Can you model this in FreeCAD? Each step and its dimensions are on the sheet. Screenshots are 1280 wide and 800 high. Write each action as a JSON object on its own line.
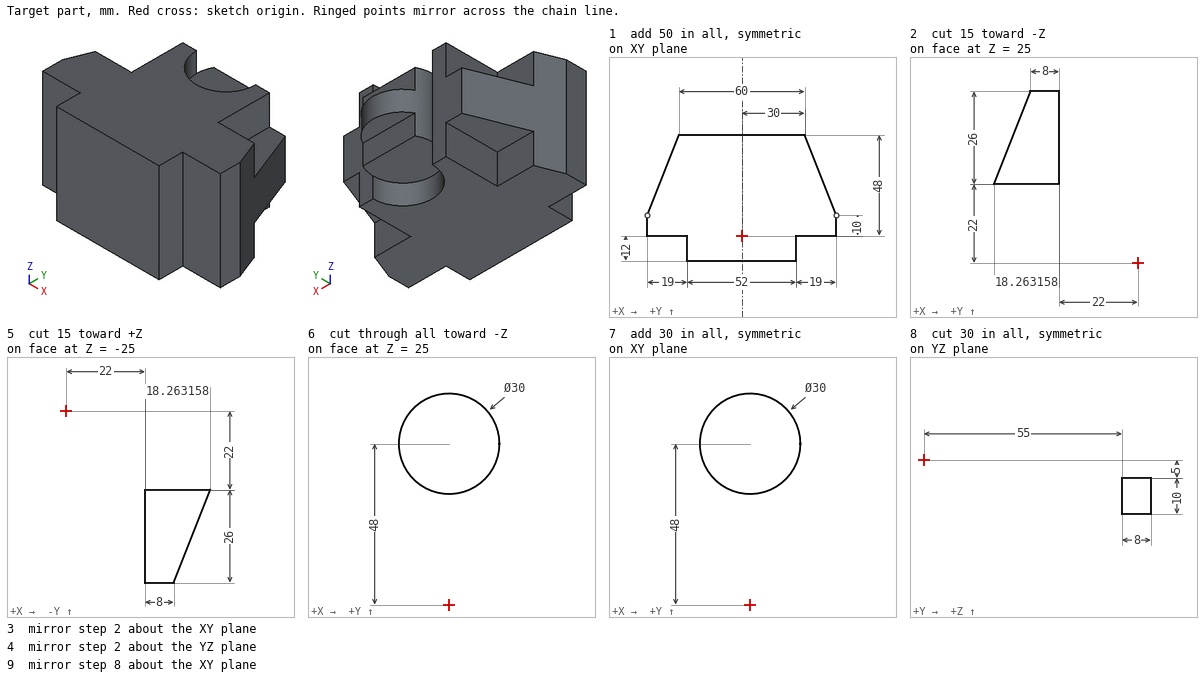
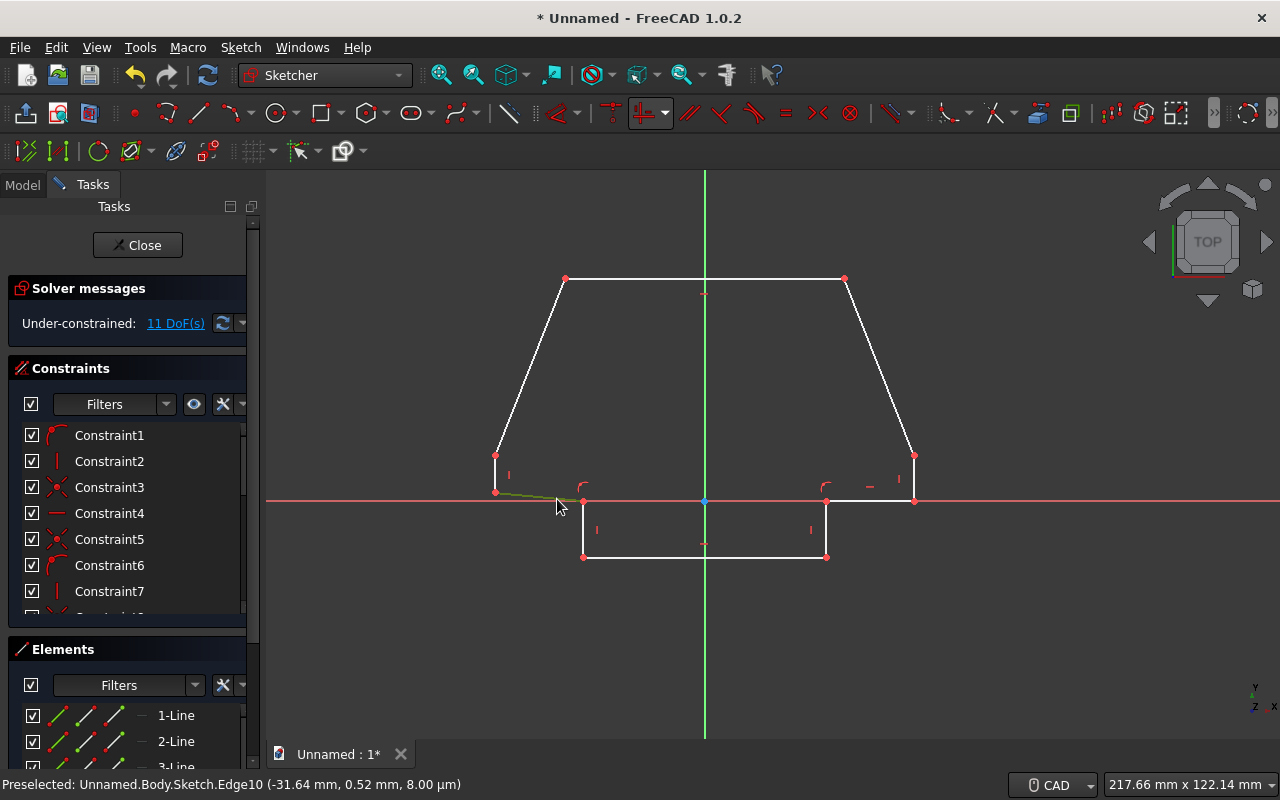
{"action": "left_click", "coordinate": [668, 114]}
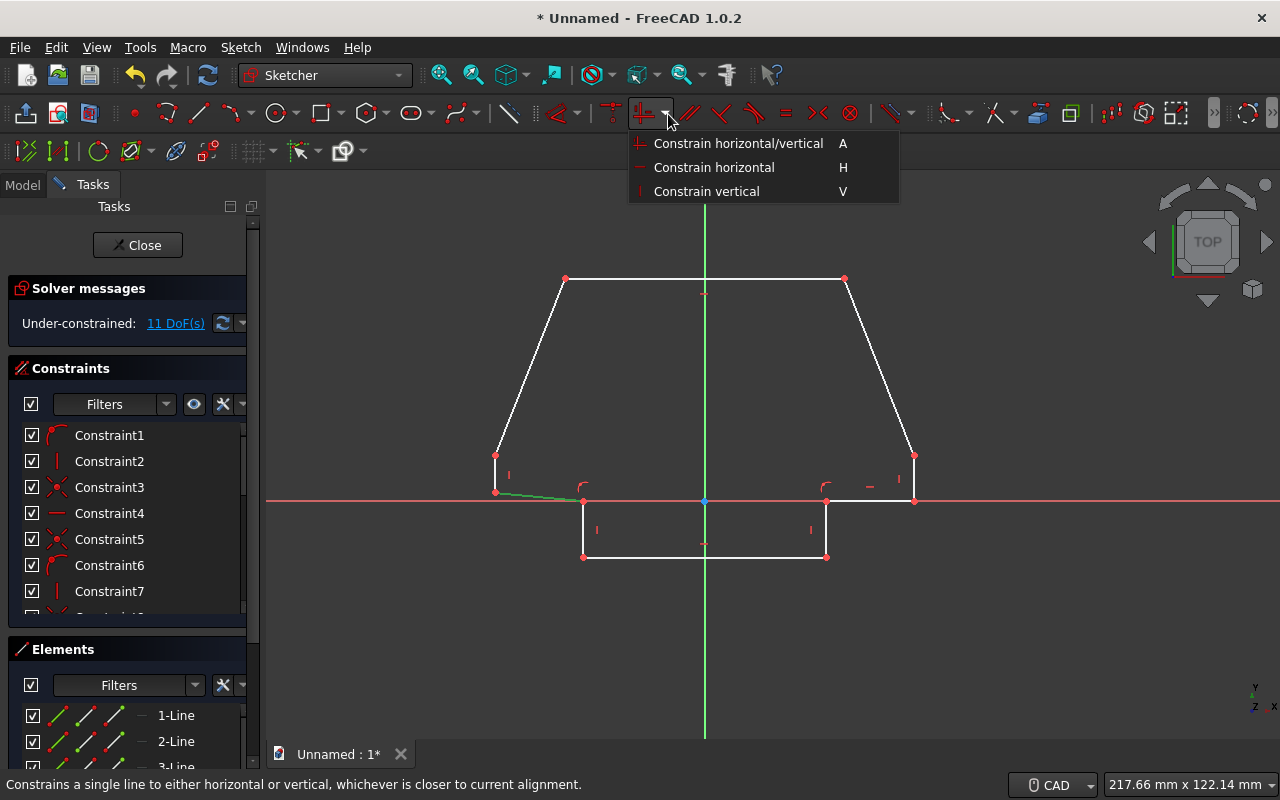
{"action": "left_click", "coordinate": [764, 167]}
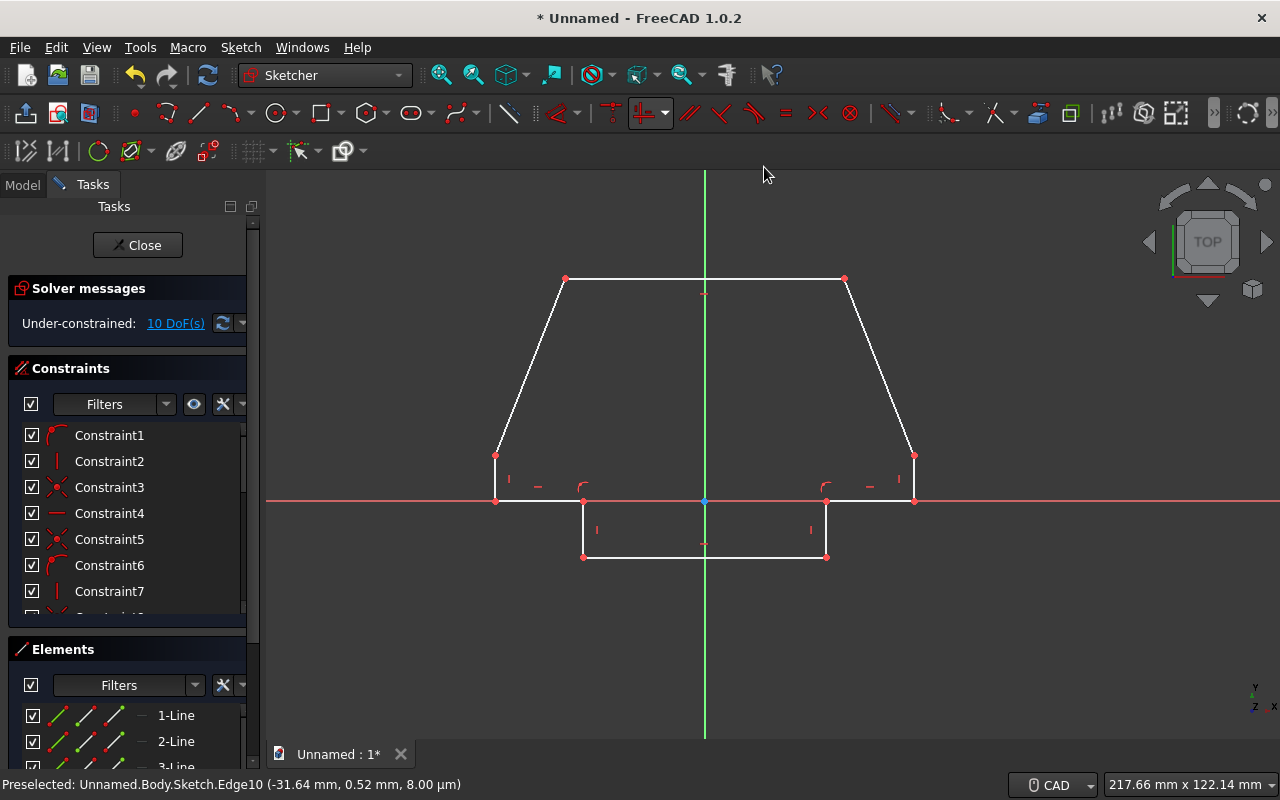
{"action": "left_click", "coordinate": [914, 456]}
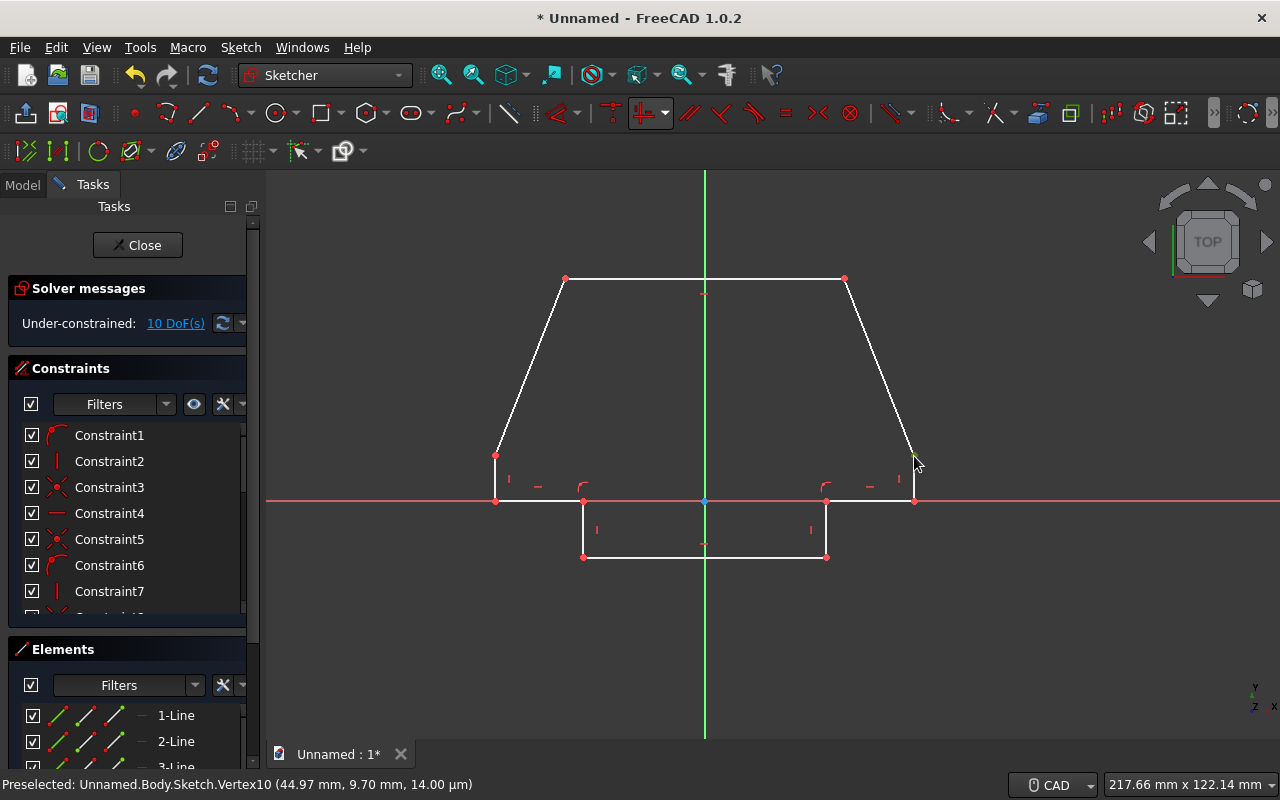
{"action": "left_click", "coordinate": [495, 456]}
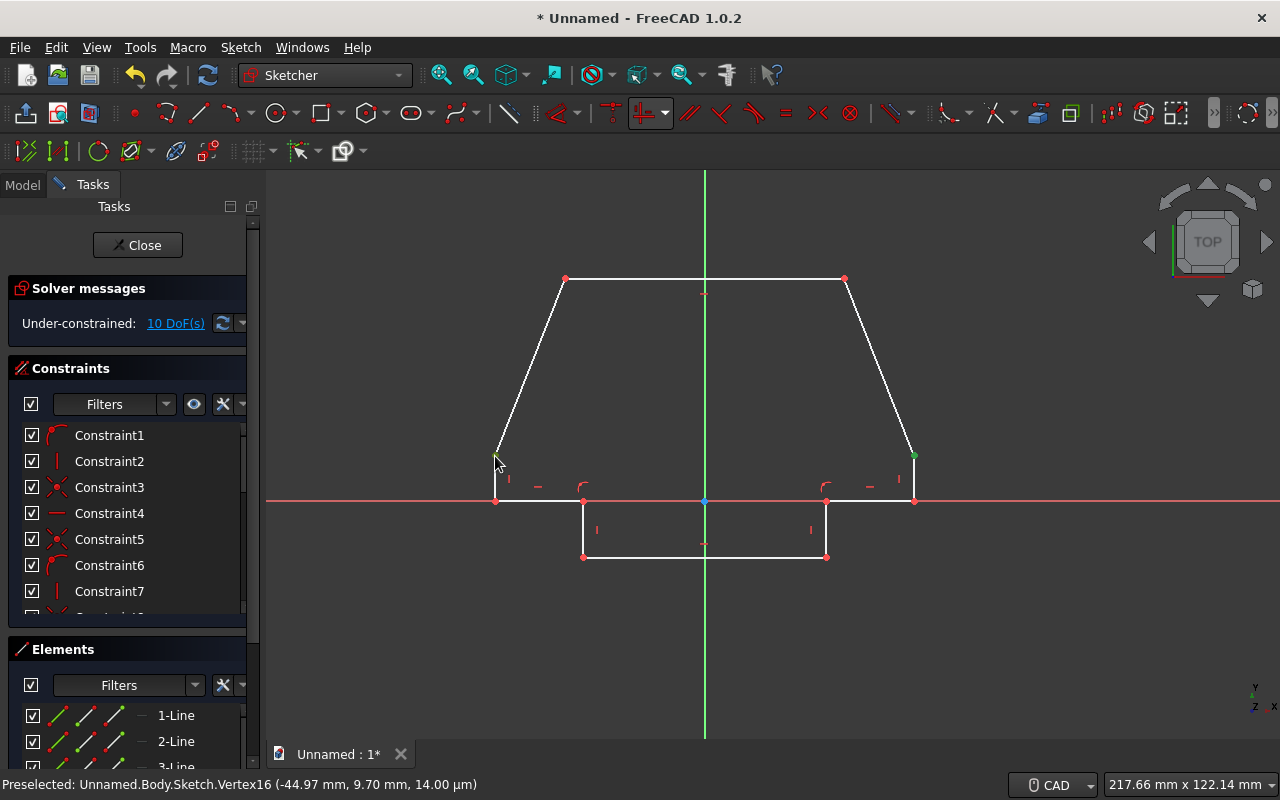
{"action": "left_click", "coordinate": [705, 674]}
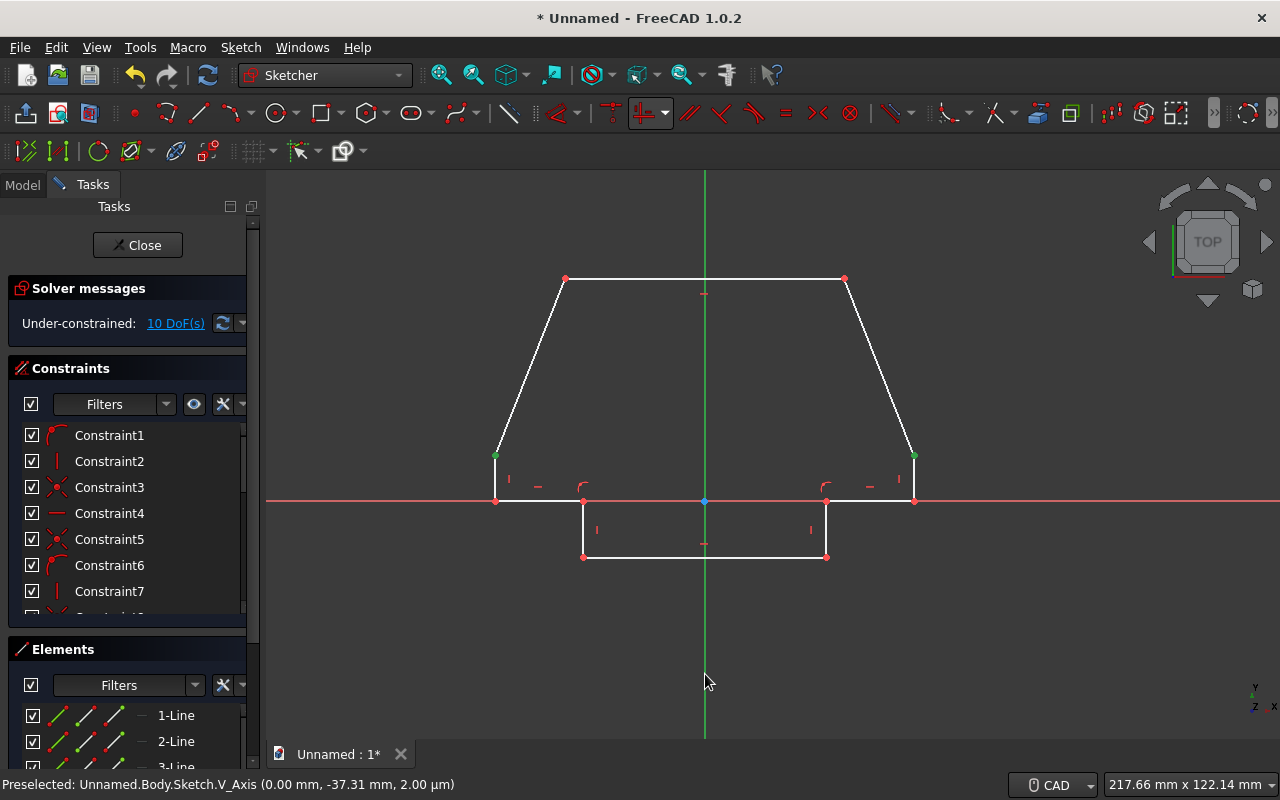
{"action": "left_click", "coordinate": [818, 114]}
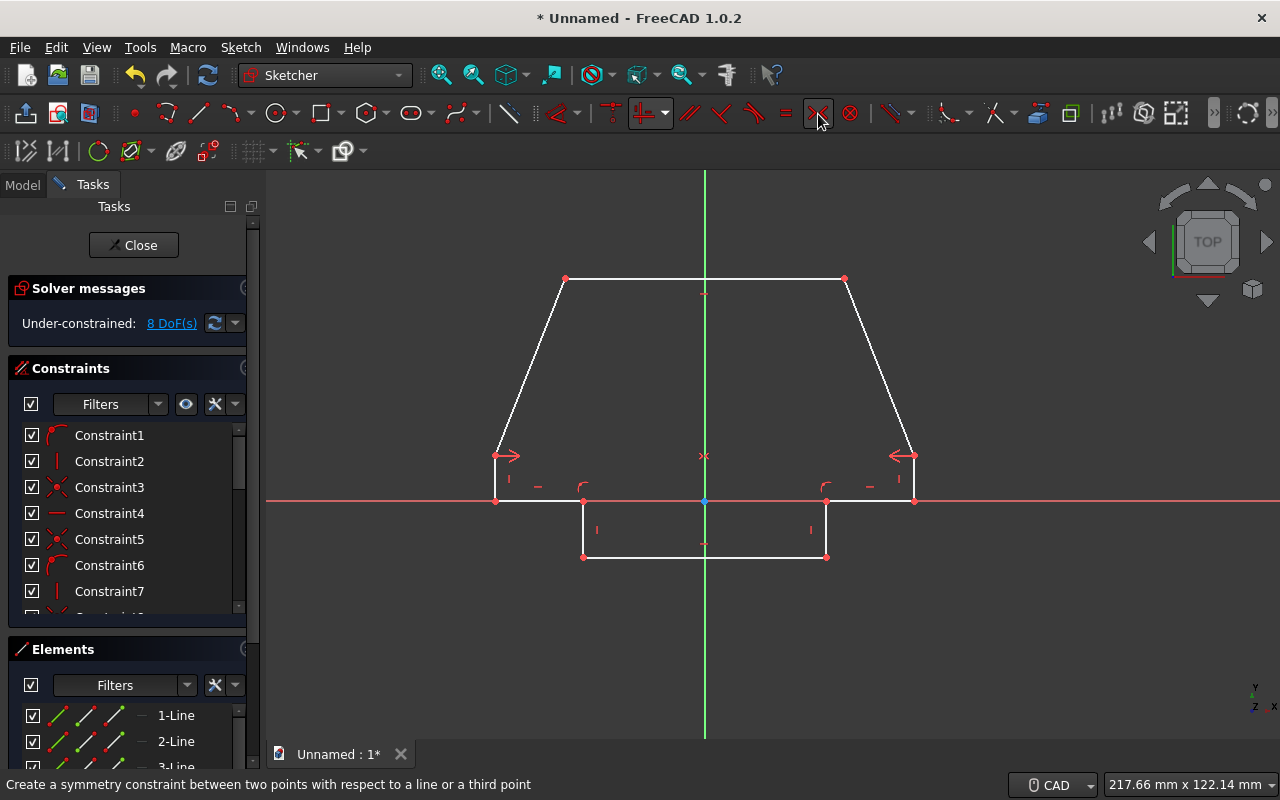
{"action": "left_click", "coordinate": [583, 518]}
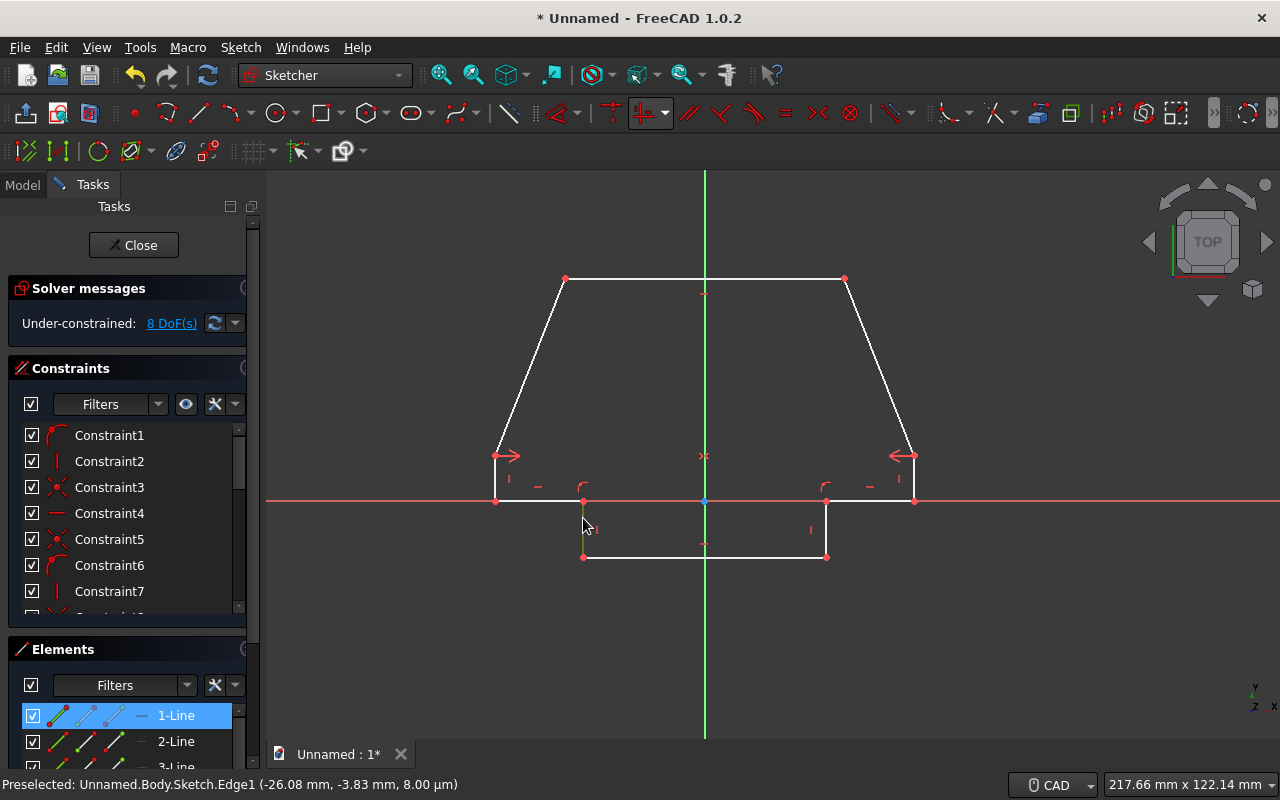
{"action": "key", "text": "i"}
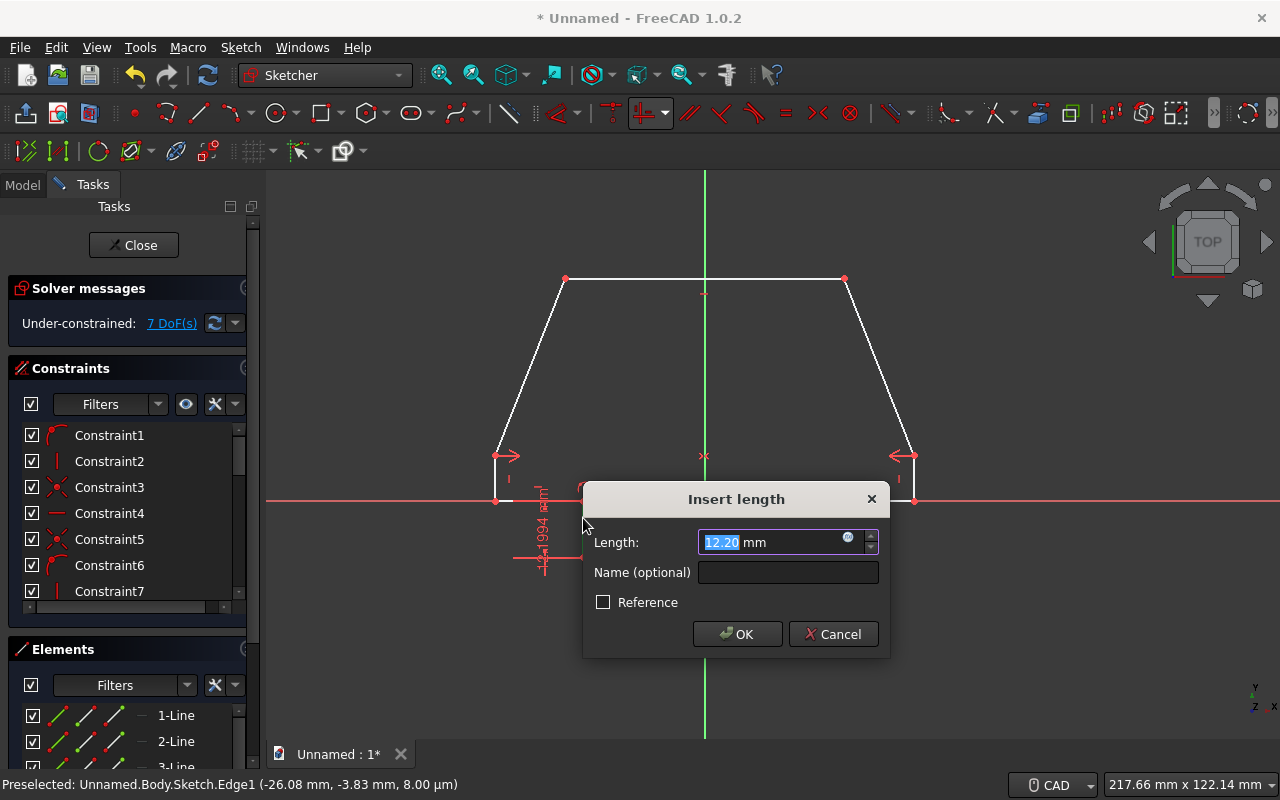
{"action": "type", "text": "12"}
{"action": "key", "text": "Return"}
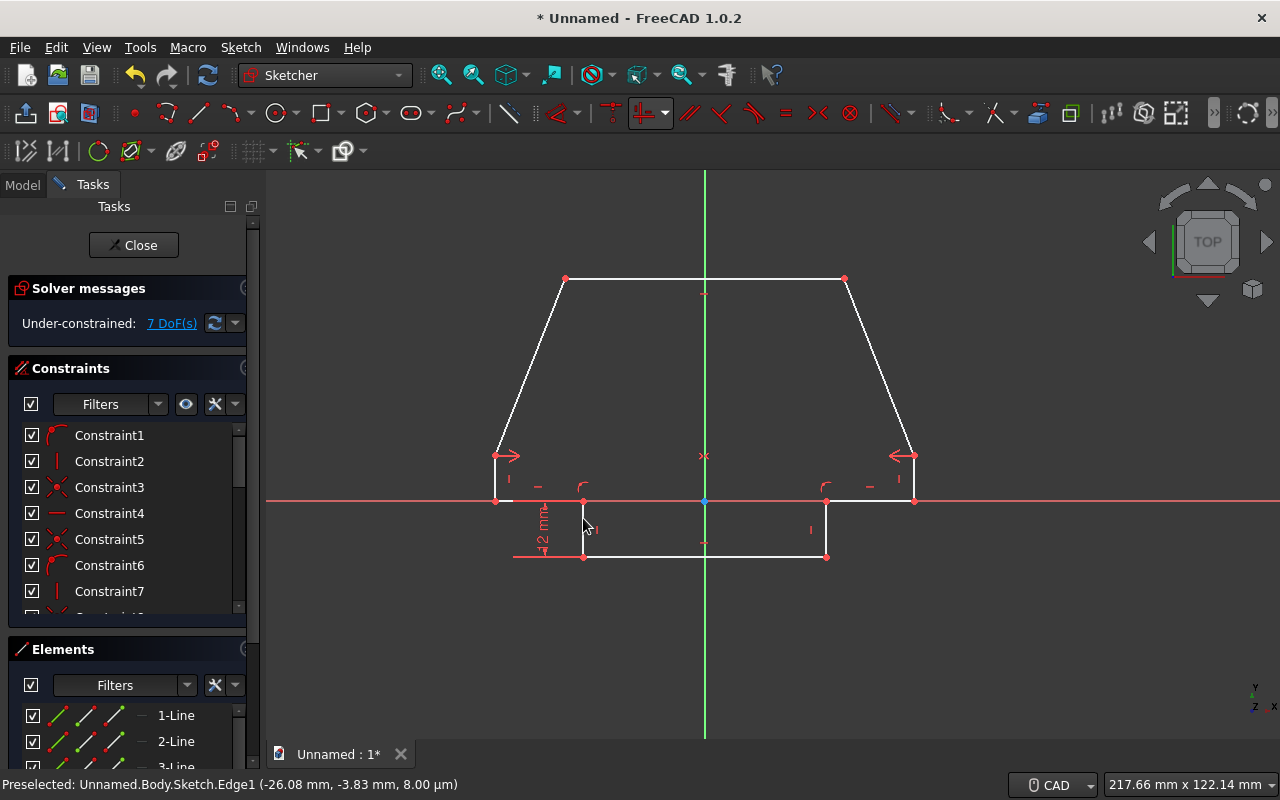
{"action": "left_click", "coordinate": [656, 557]}